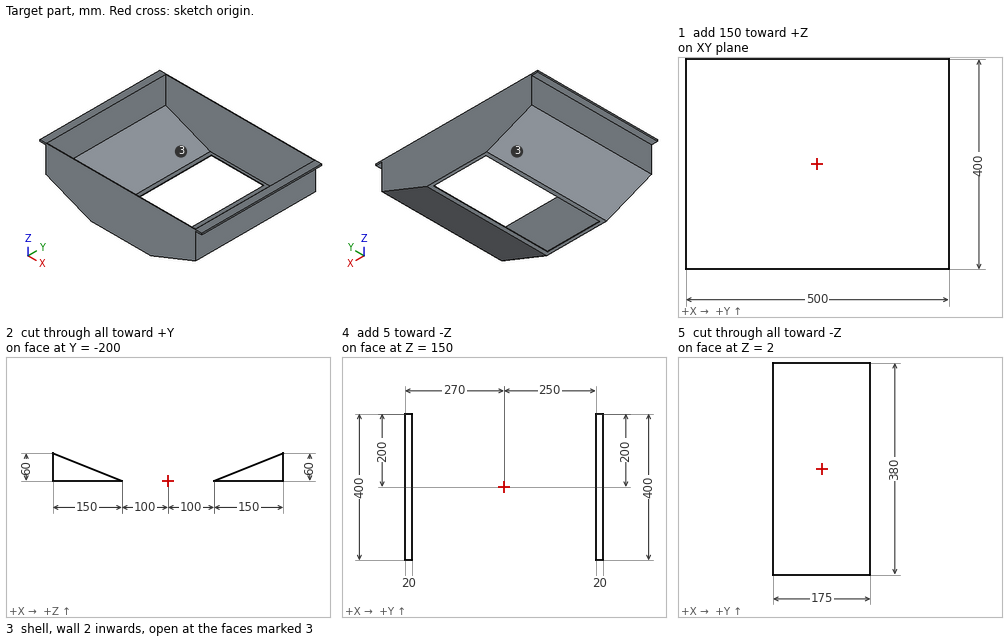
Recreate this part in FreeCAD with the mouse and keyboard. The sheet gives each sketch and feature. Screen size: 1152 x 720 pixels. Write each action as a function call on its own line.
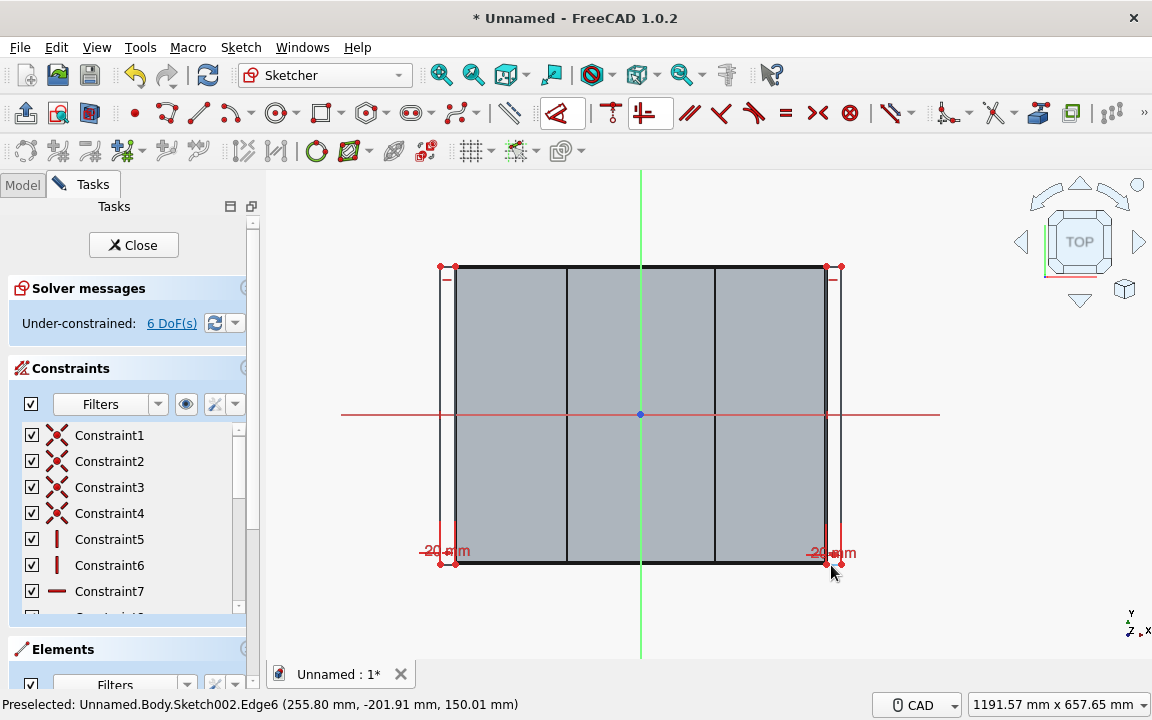
click(440, 356)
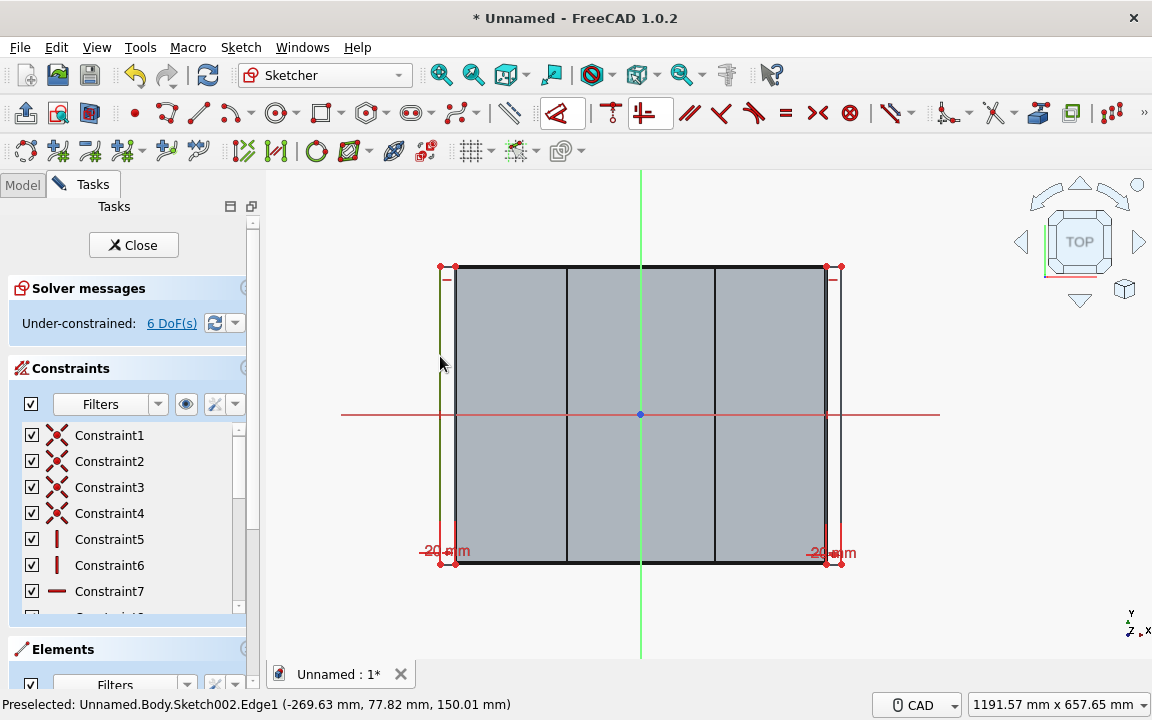
key(i)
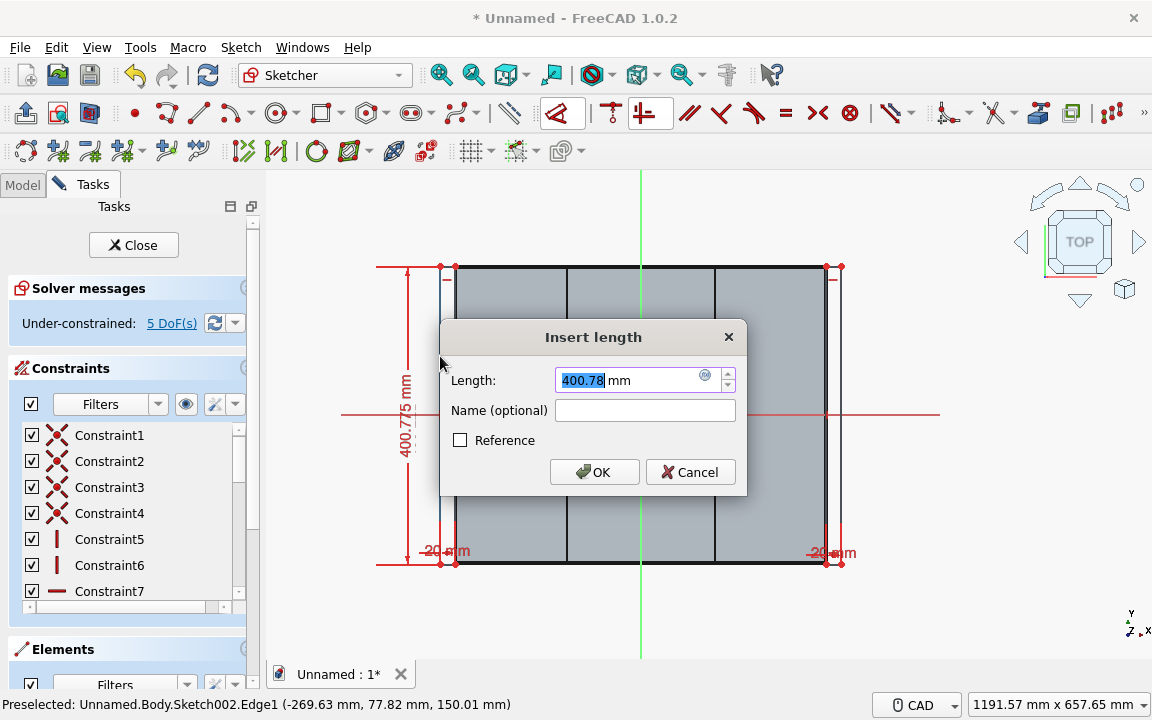
text(400)
key(Return)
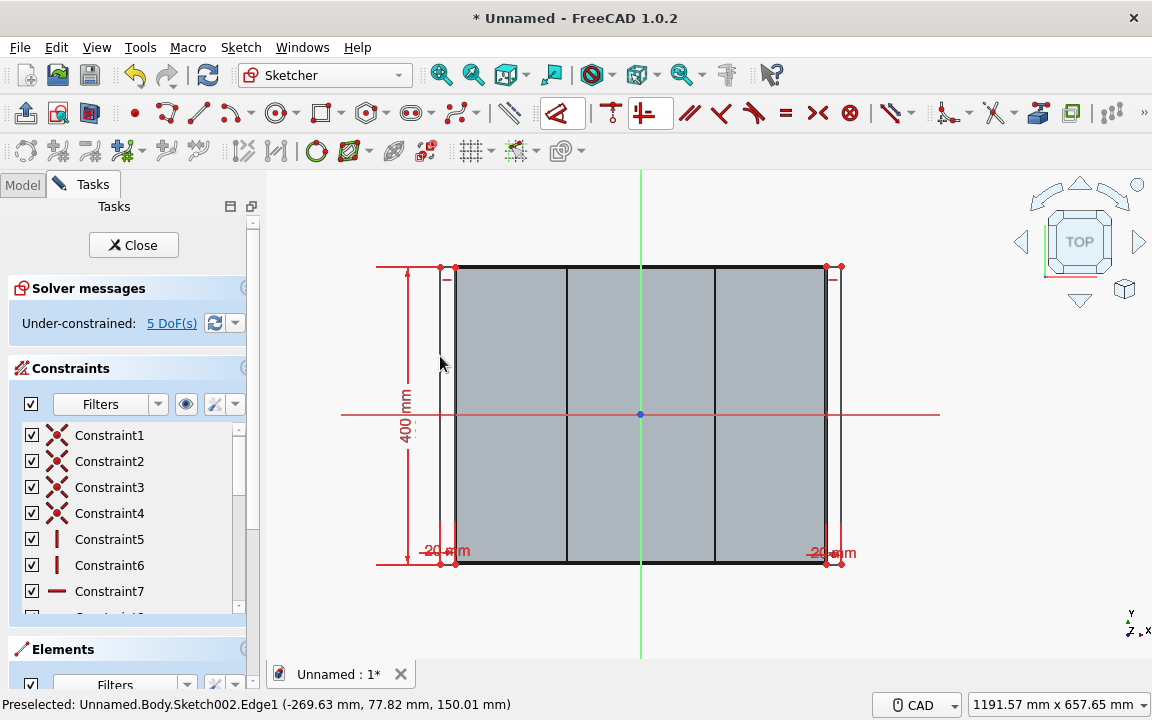
click(826, 356)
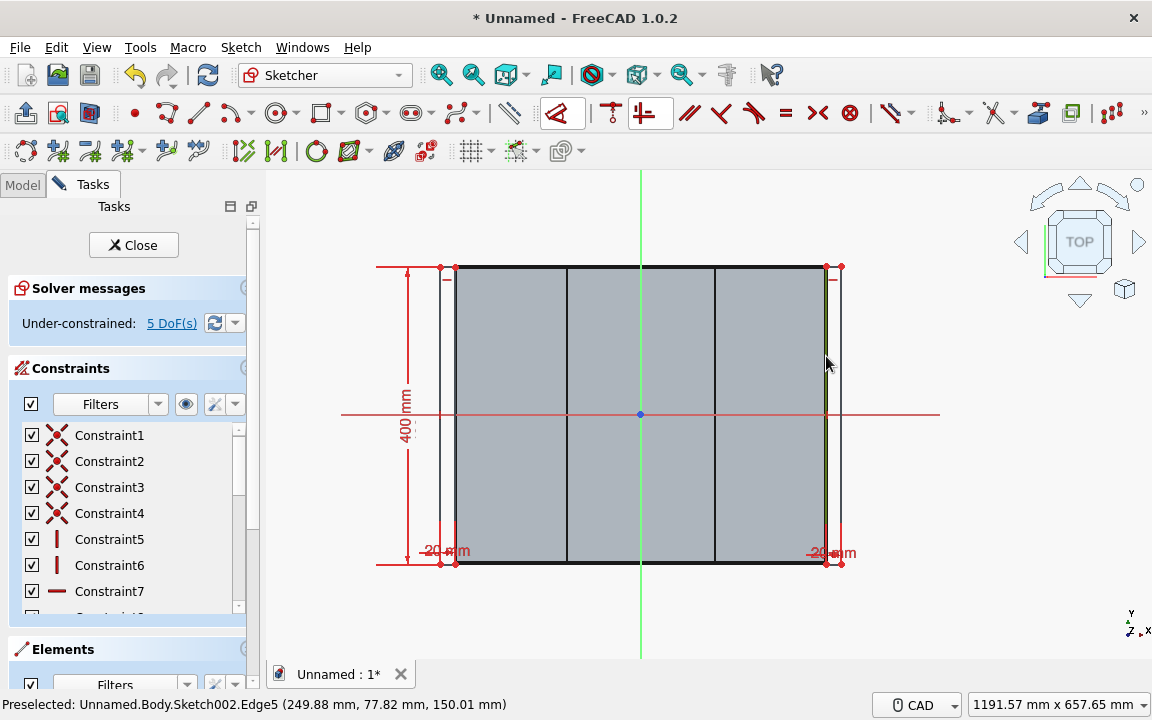
click(580, 114)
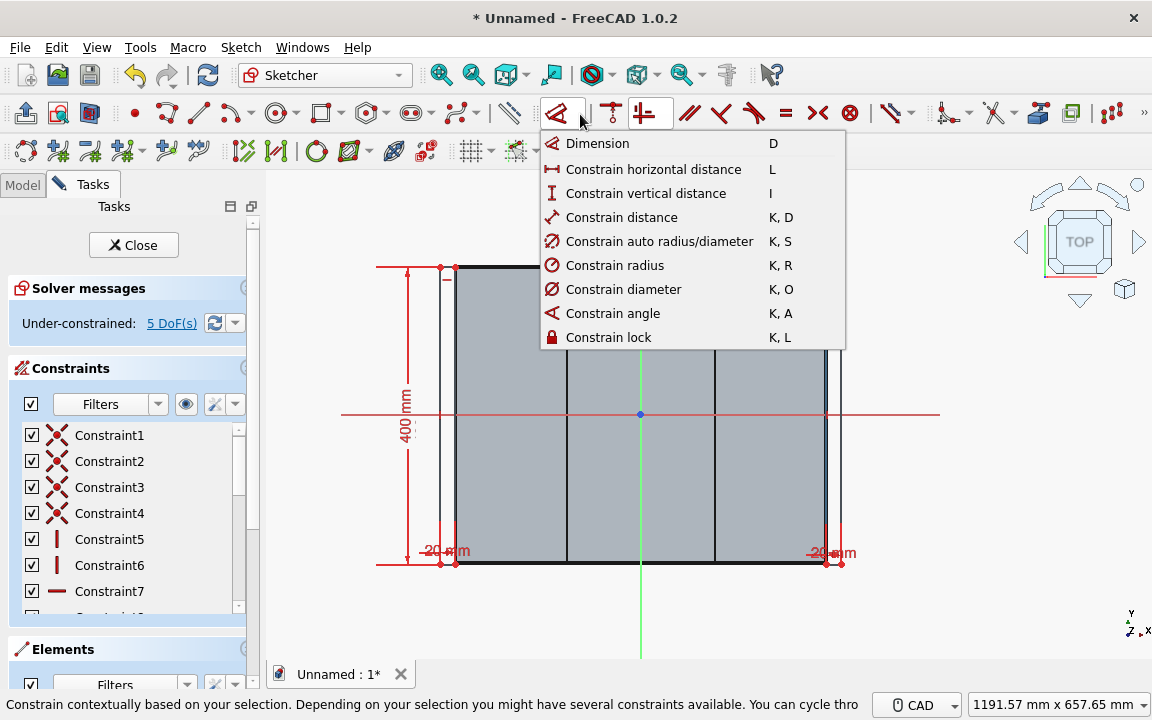
click(693, 193)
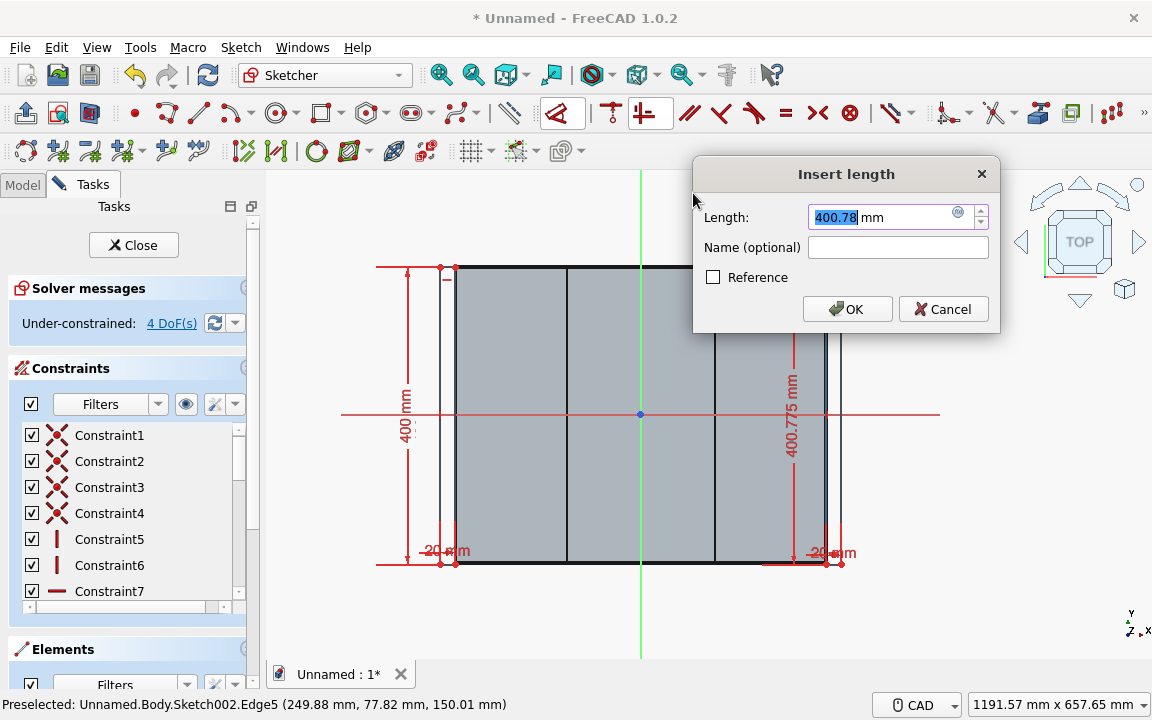
text(400)
key(Return)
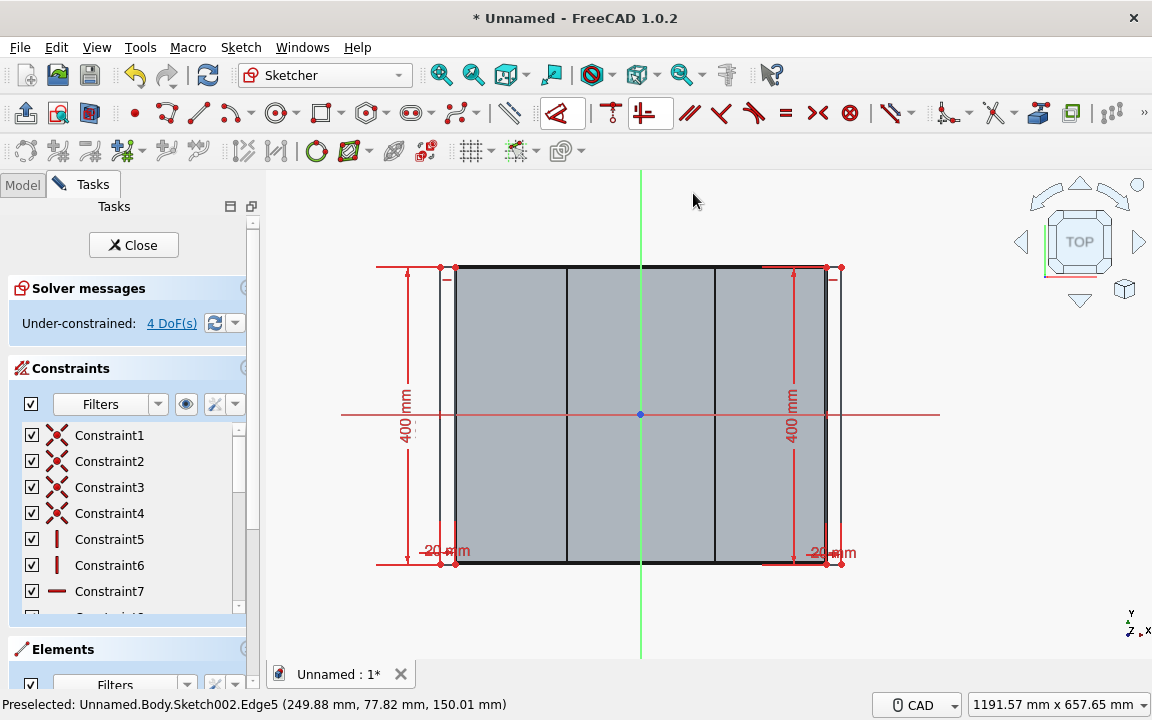
click(440, 267)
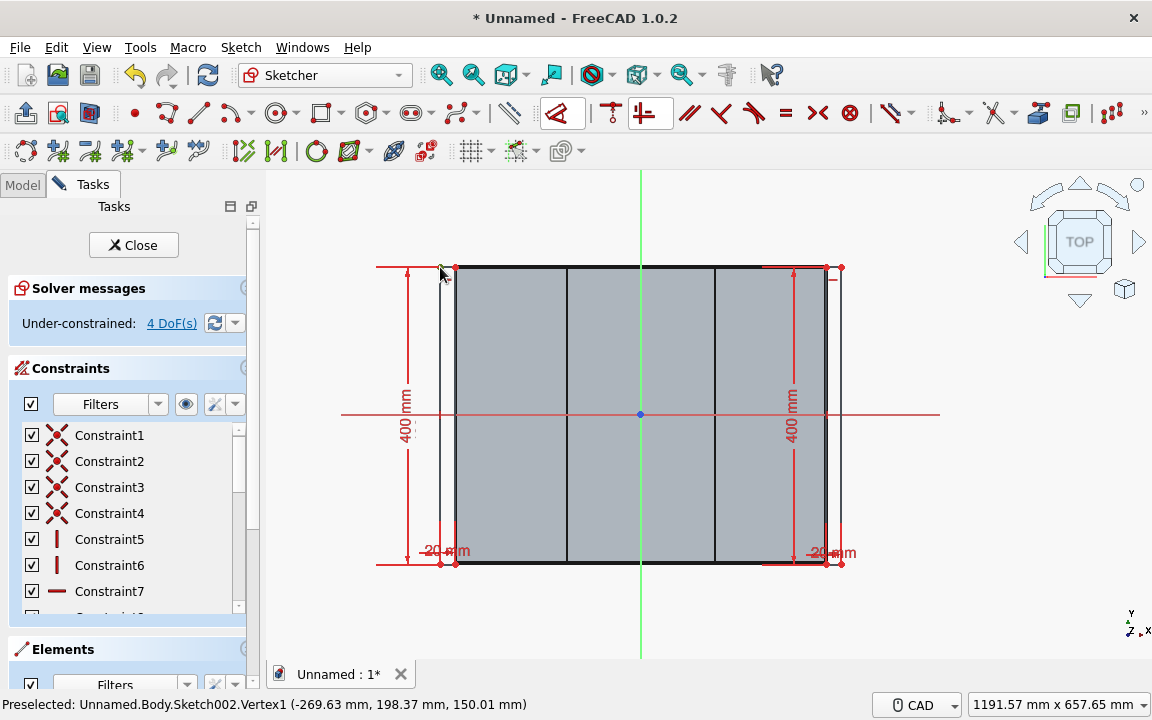
key(l)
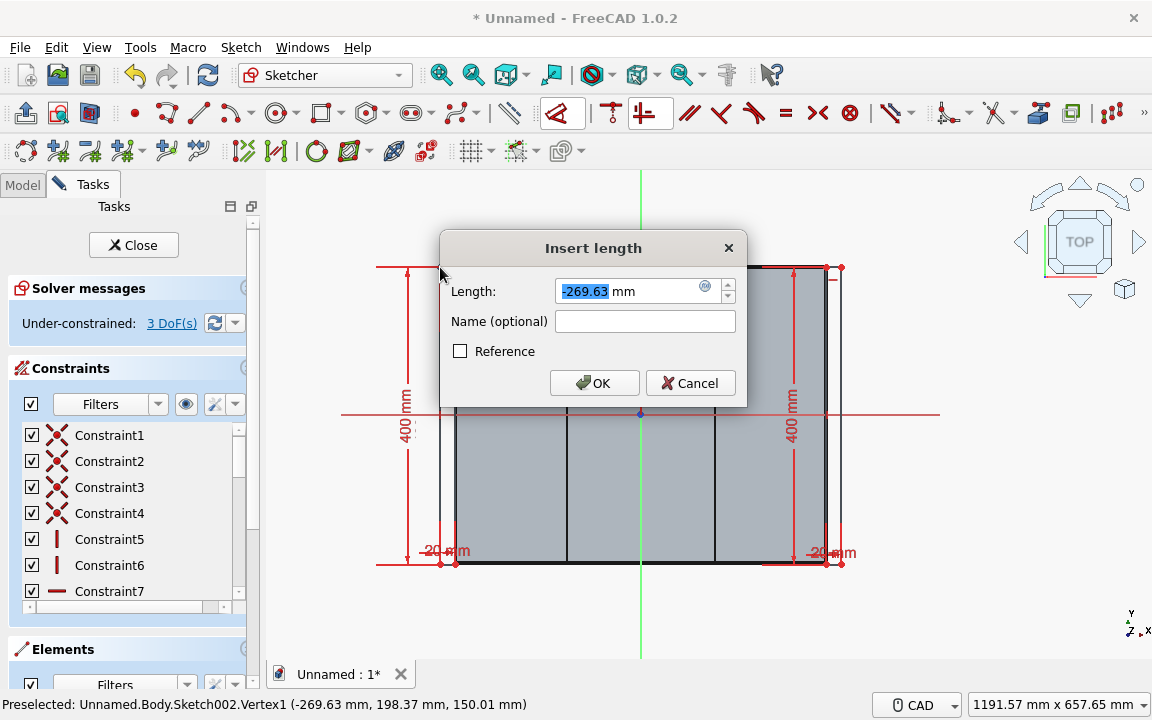
text(-270)
key(Return)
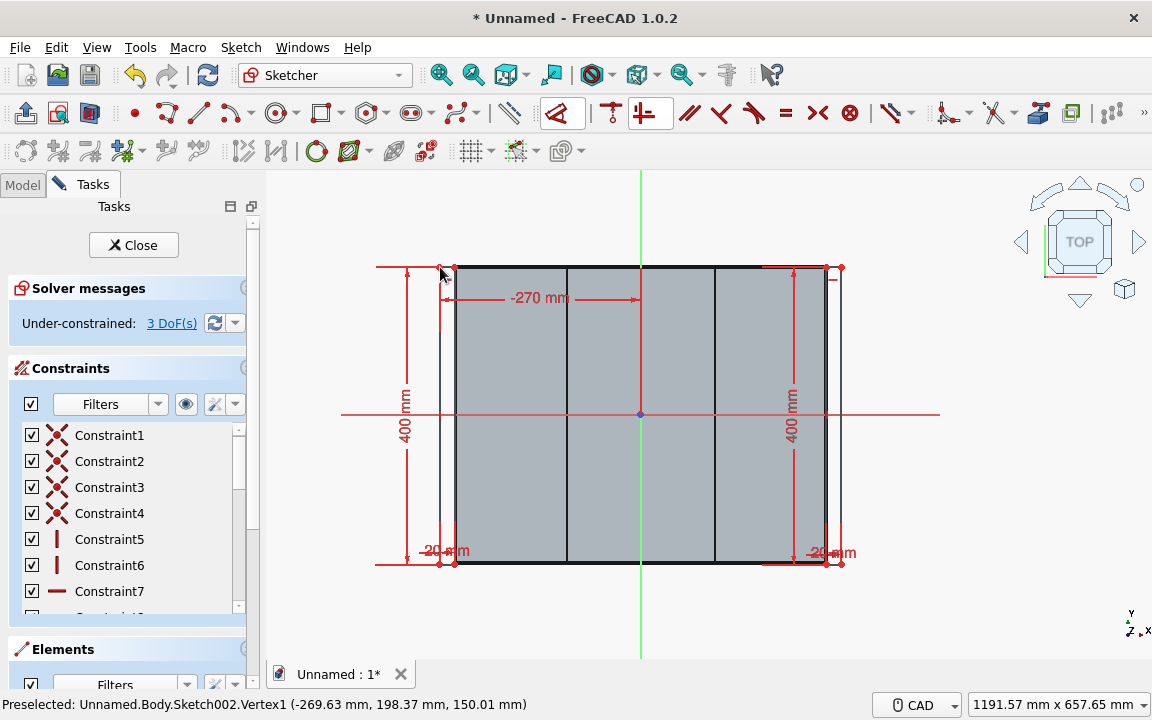
click(440, 267)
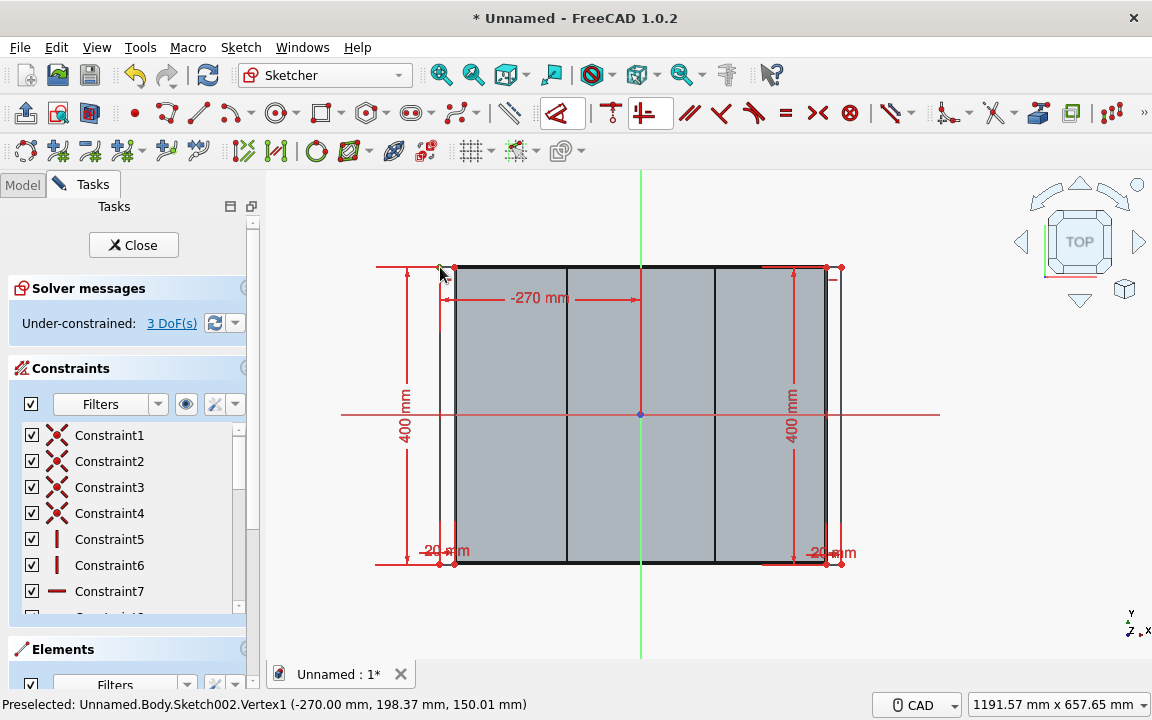
click(580, 114)